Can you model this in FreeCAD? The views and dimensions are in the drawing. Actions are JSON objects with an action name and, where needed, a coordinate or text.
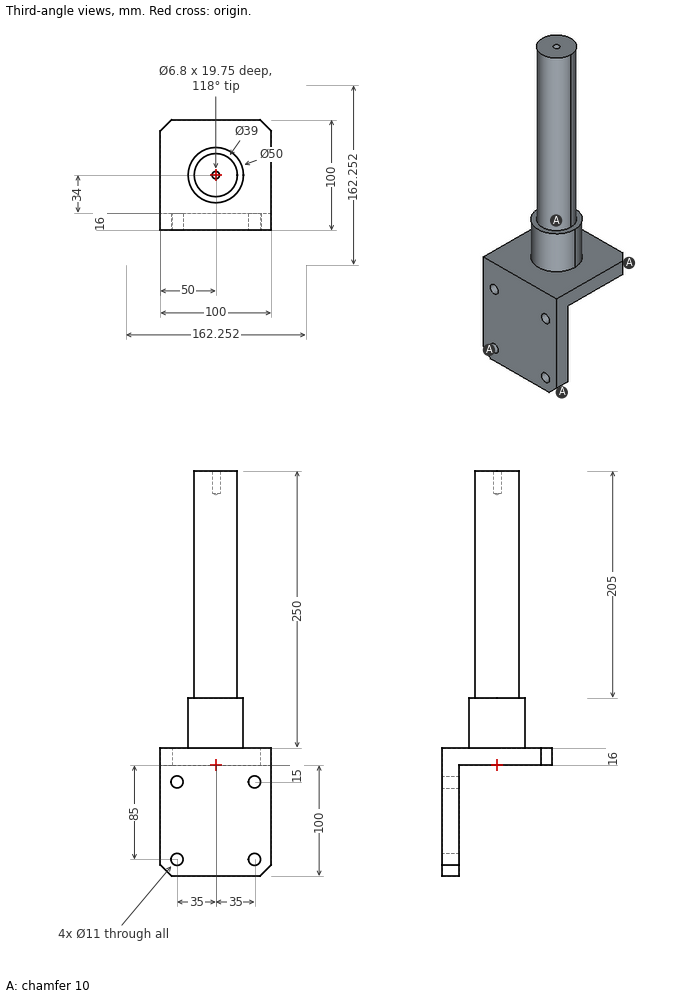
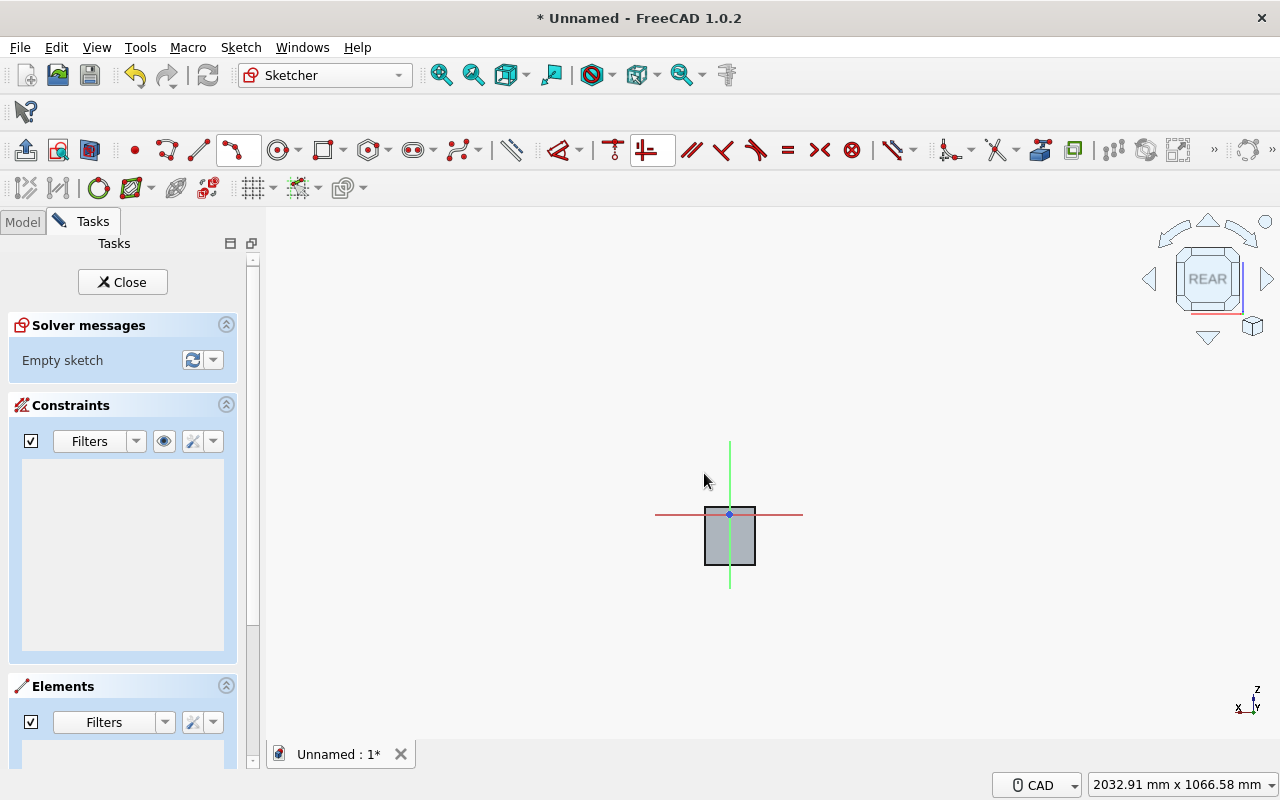
{"action": "scroll", "coordinate": [734, 547], "scroll_direction": "up", "scroll_amount": 10}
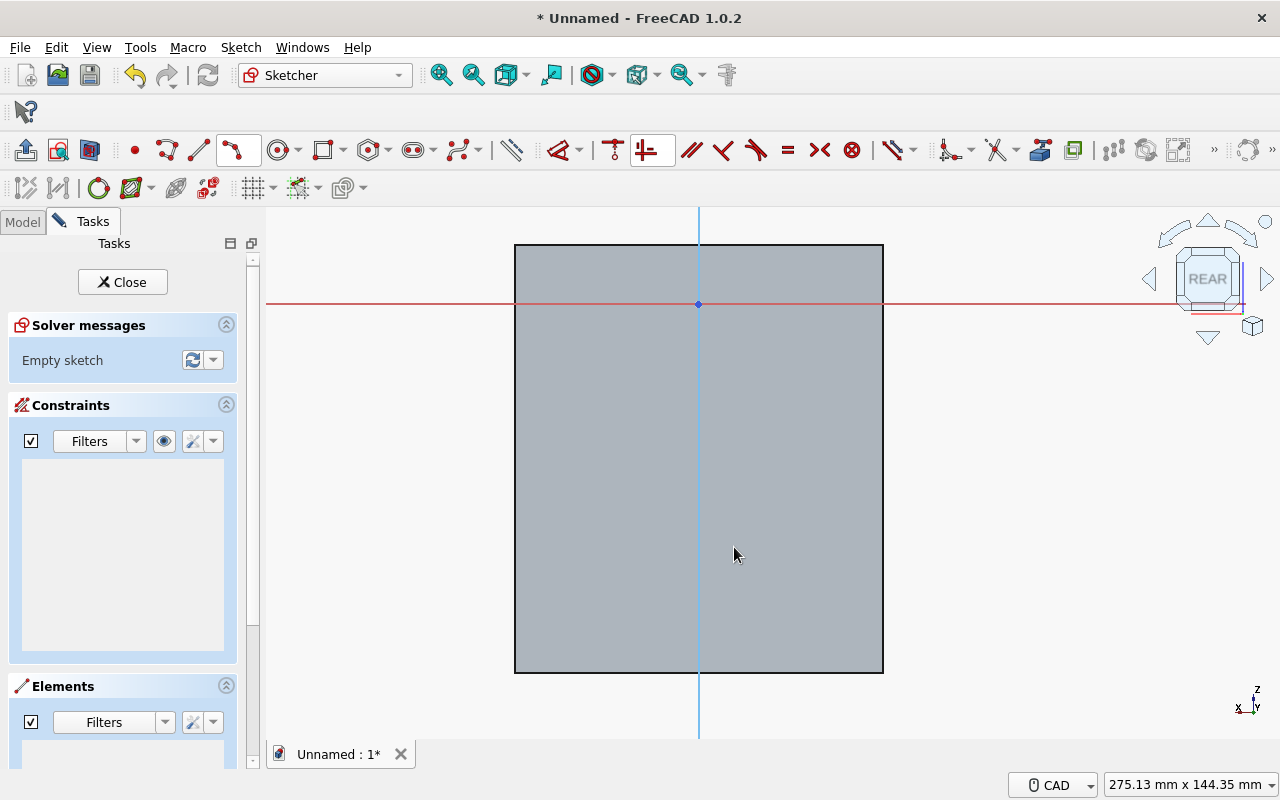
{"action": "key", "text": "g c"}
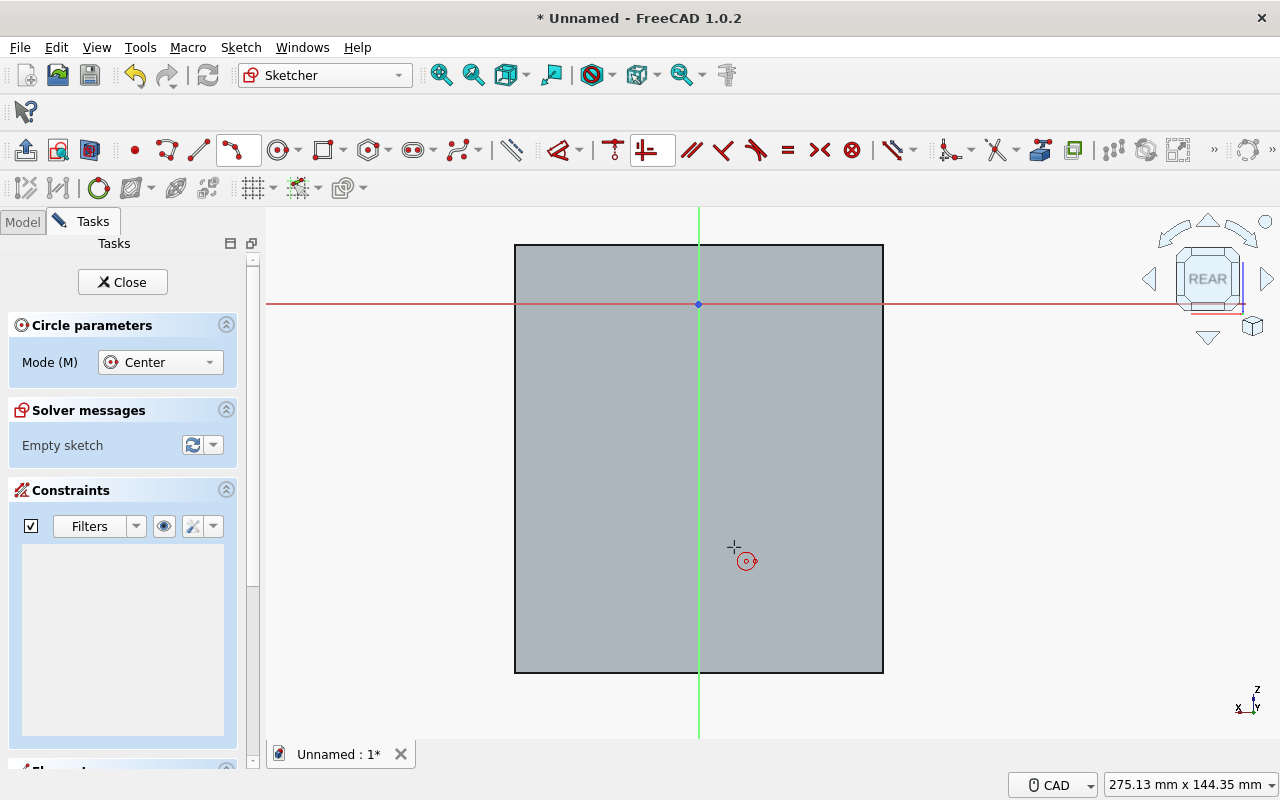
{"action": "left_click", "coordinate": [828, 618]}
{"action": "left_click", "coordinate": [842, 603]}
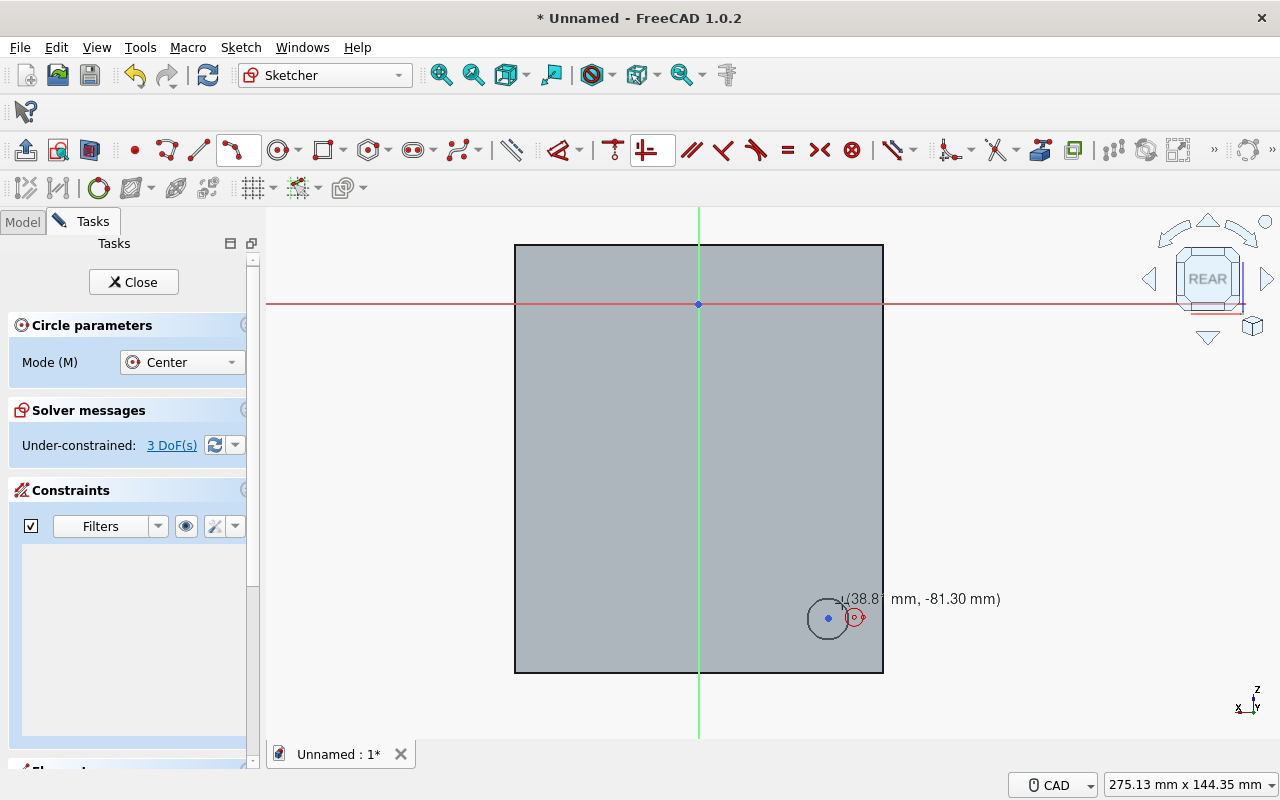
{"action": "left_click", "coordinate": [570, 618]}
{"action": "left_click", "coordinate": [584, 603]}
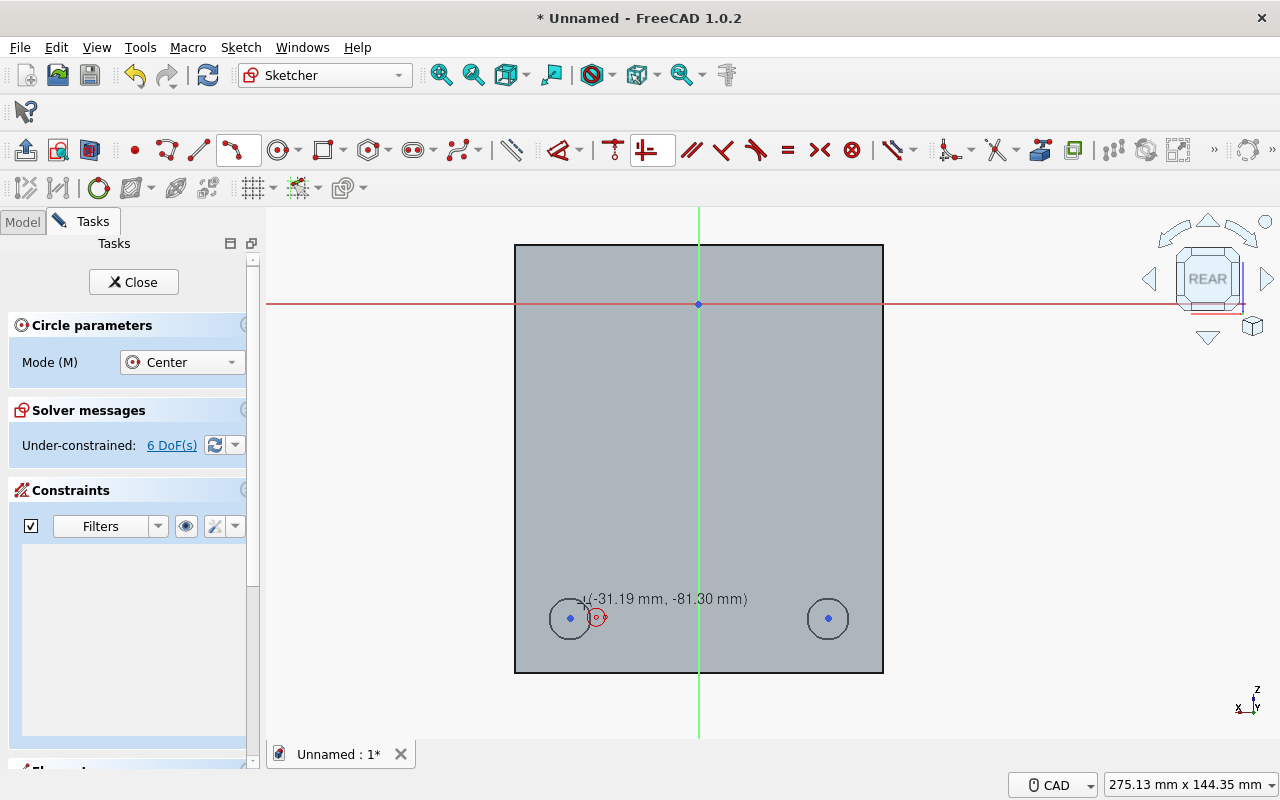
{"action": "left_click", "coordinate": [570, 360]}
{"action": "left_click", "coordinate": [584, 345]}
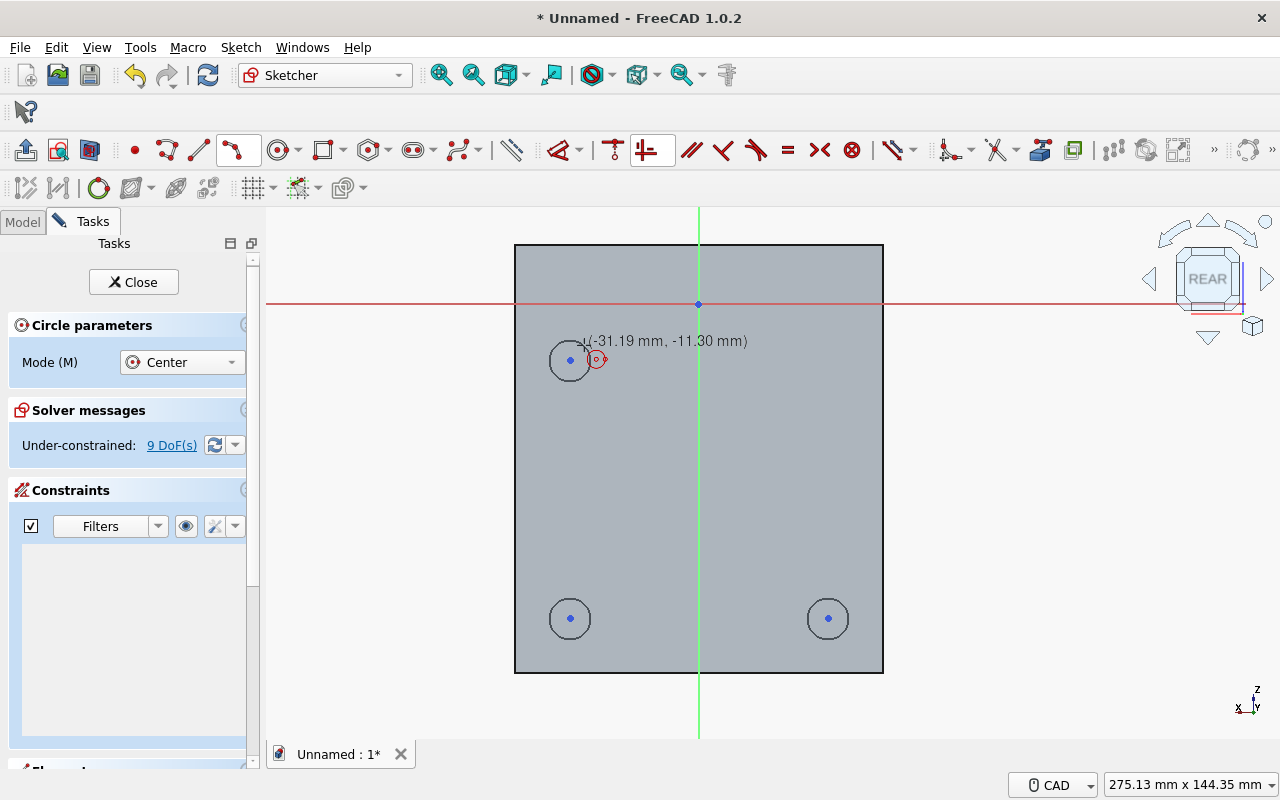
{"action": "left_click", "coordinate": [828, 360]}
{"action": "left_click", "coordinate": [842, 345]}
{"action": "key", "text": "Escape"}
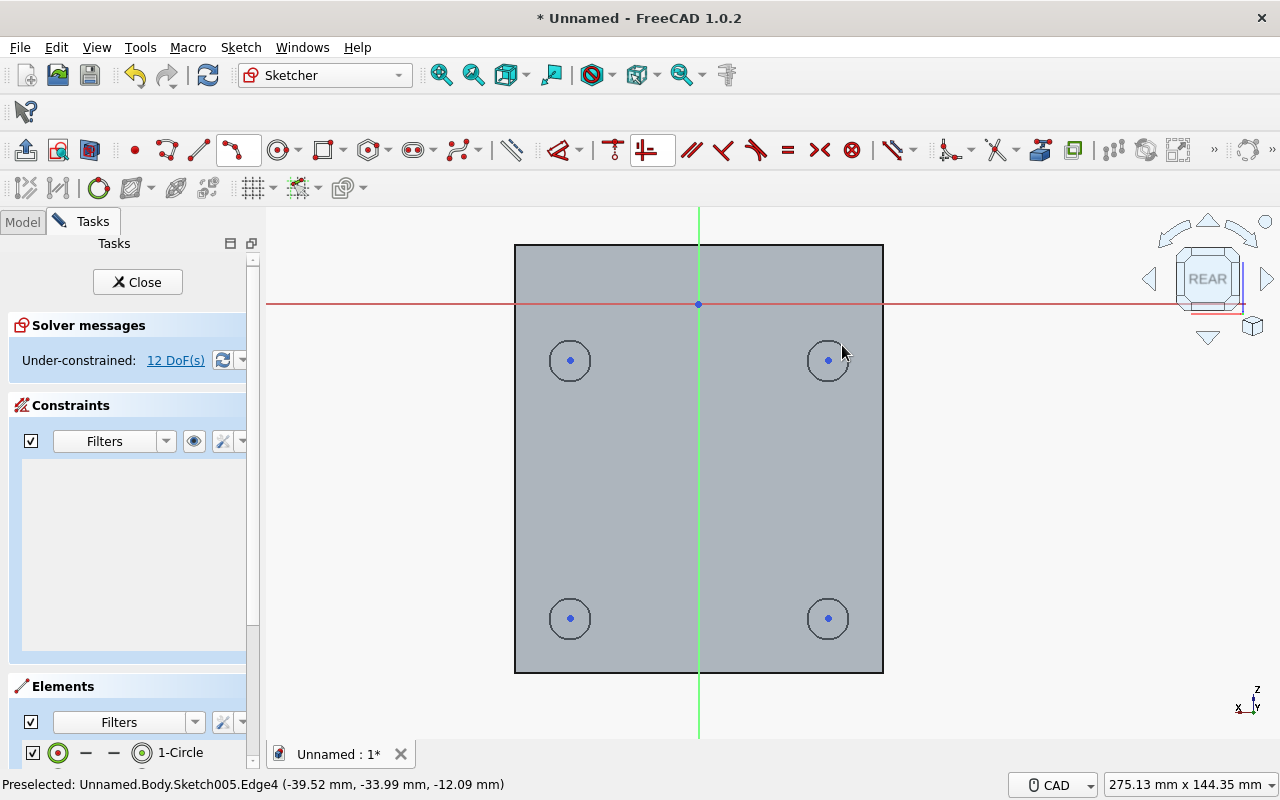
{"action": "left_click", "coordinate": [842, 604]}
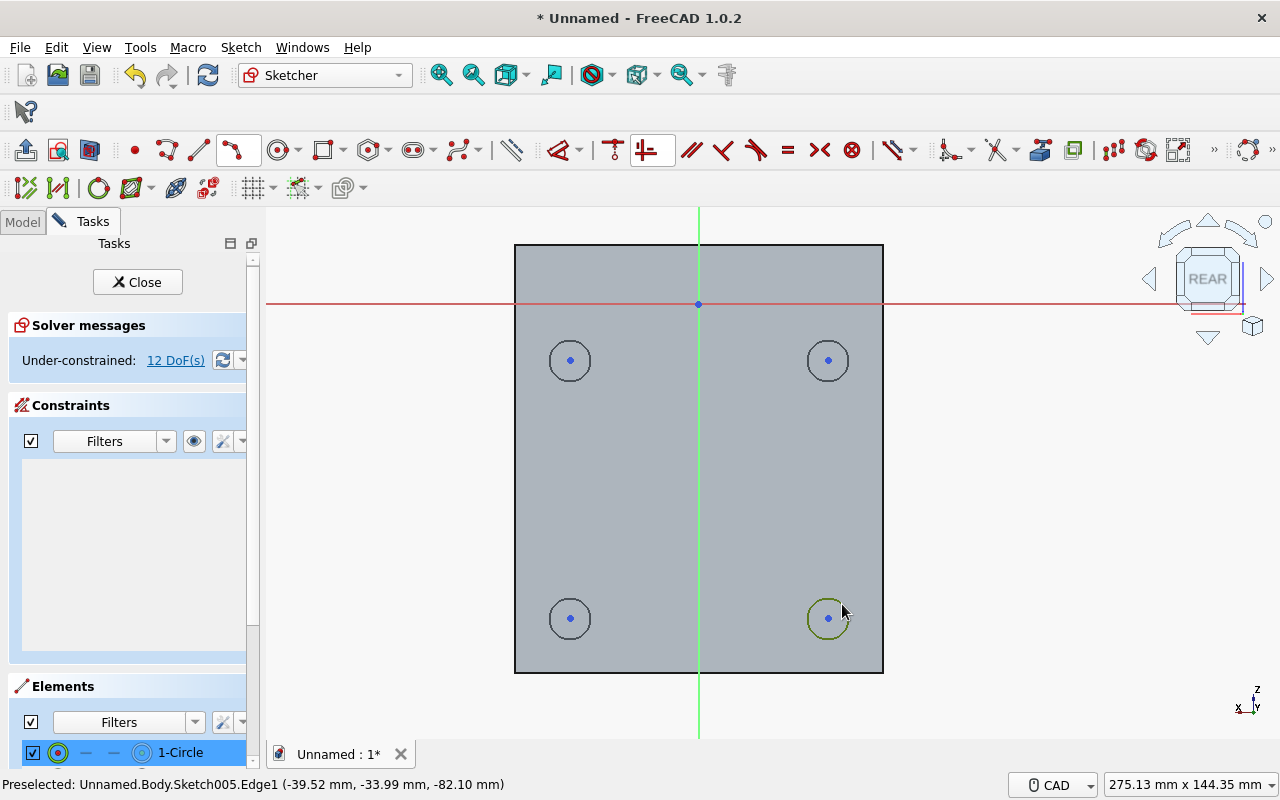
{"action": "left_click", "coordinate": [584, 604]}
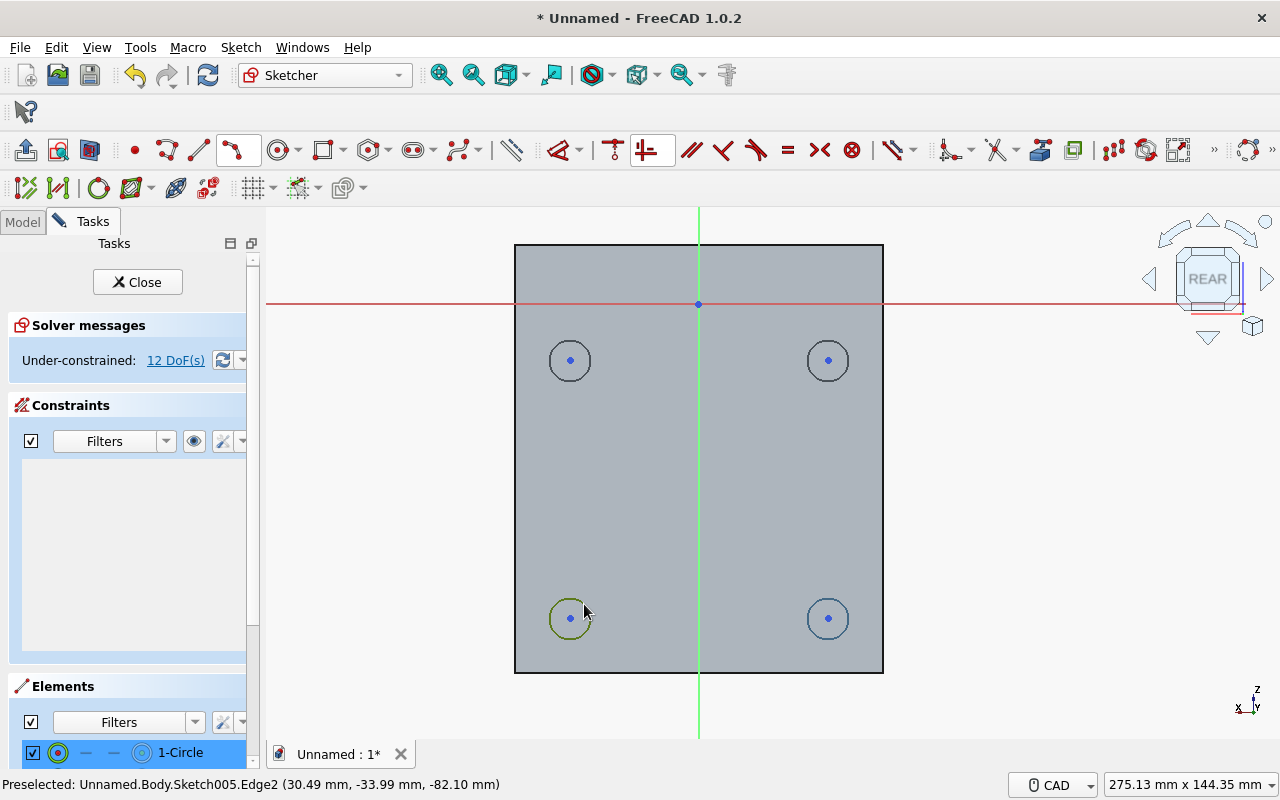
{"action": "left_click", "coordinate": [584, 346]}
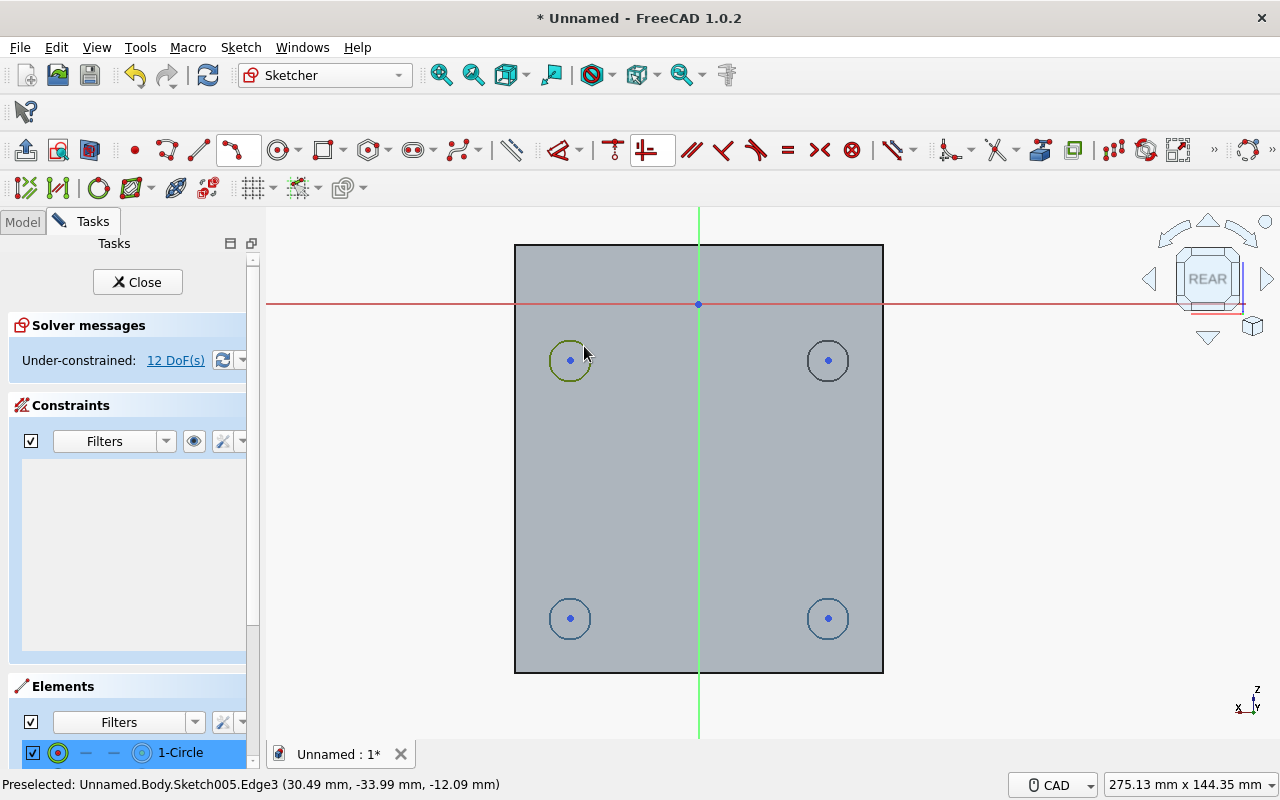
{"action": "left_click", "coordinate": [842, 346]}